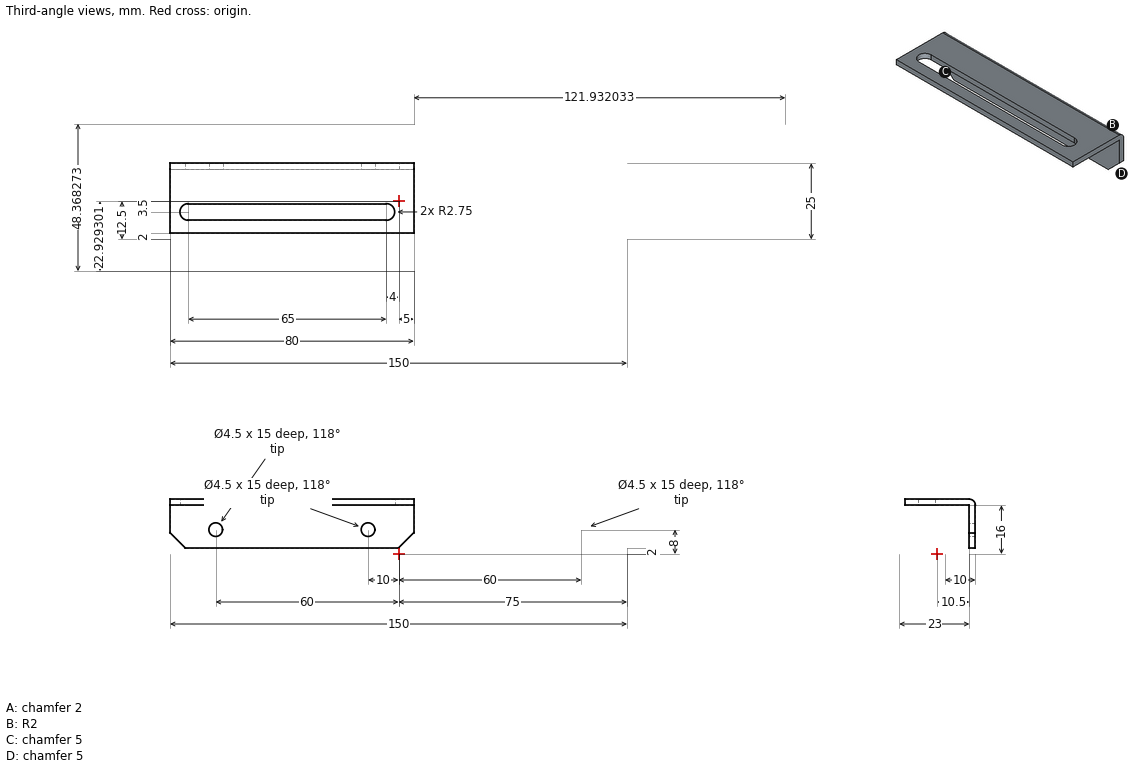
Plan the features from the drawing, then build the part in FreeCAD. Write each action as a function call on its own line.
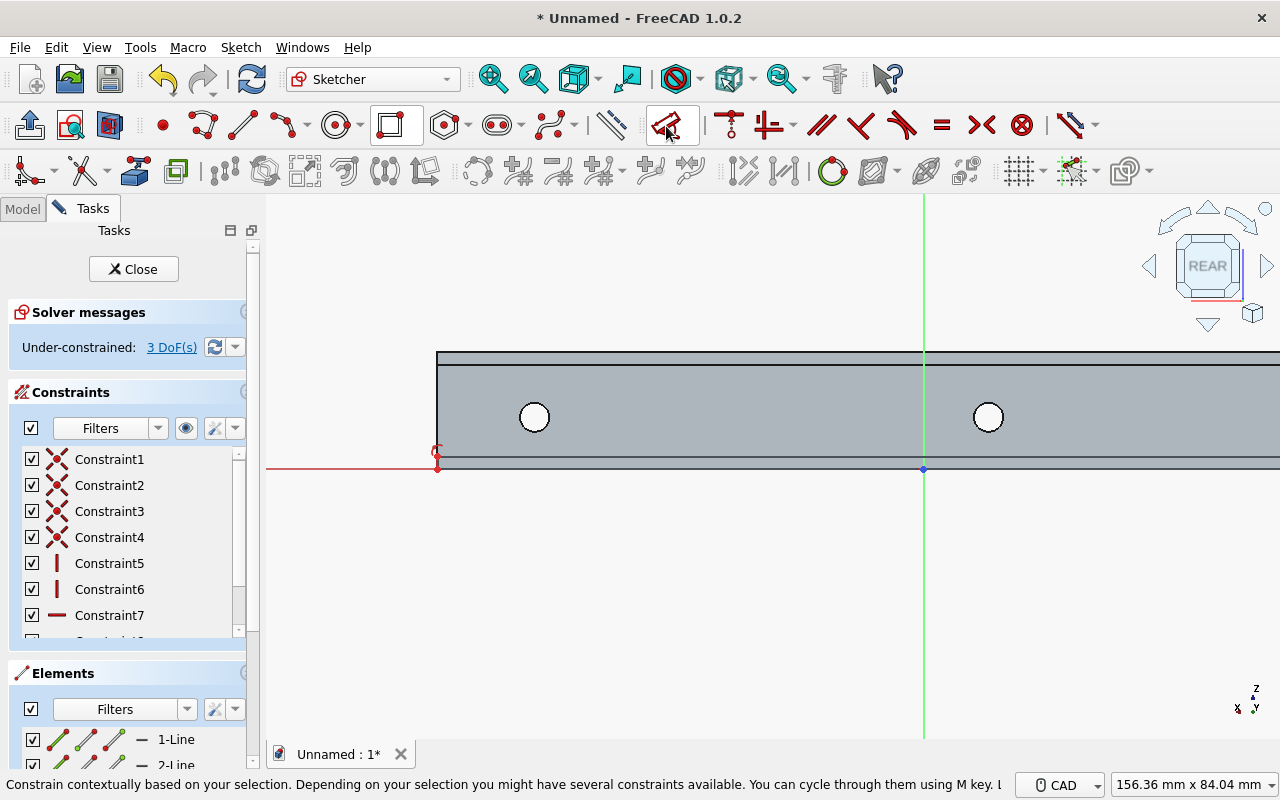
scroll(438, 463, up, 6)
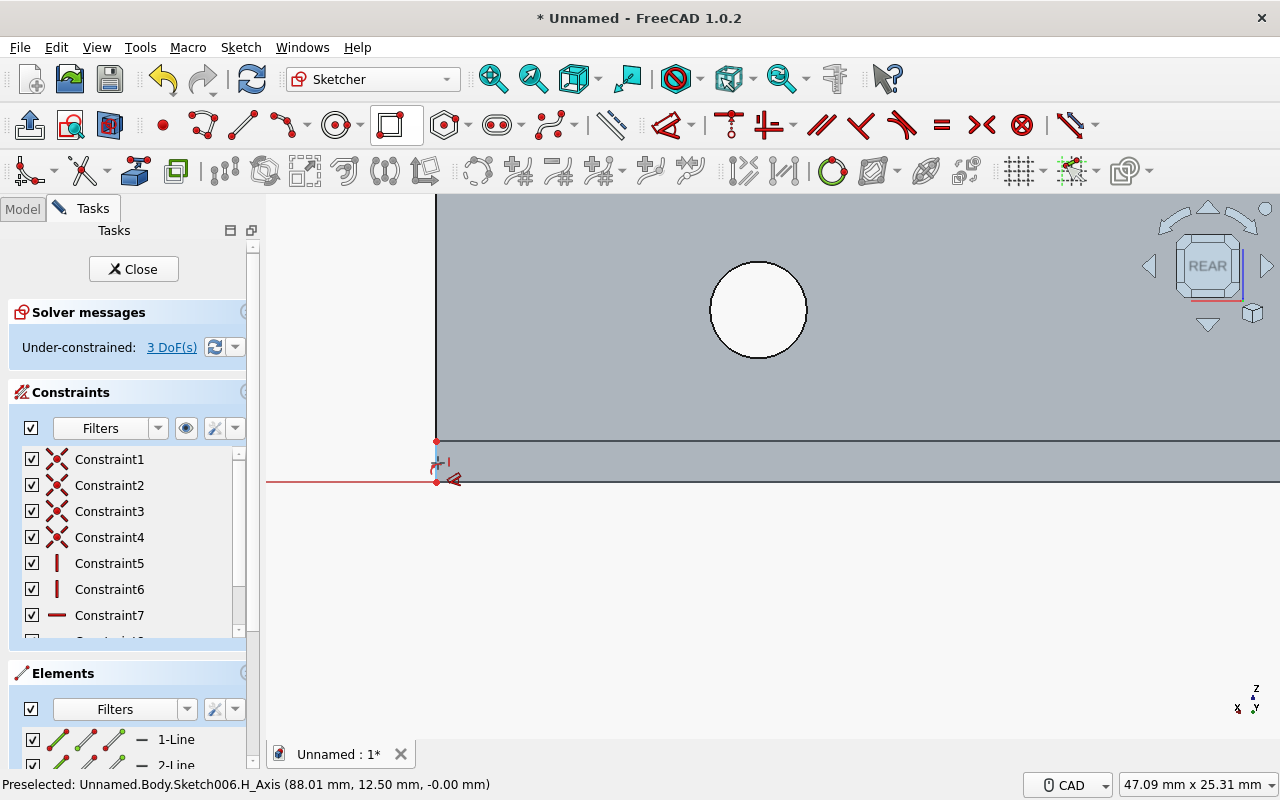
click(436, 462)
click(402, 462)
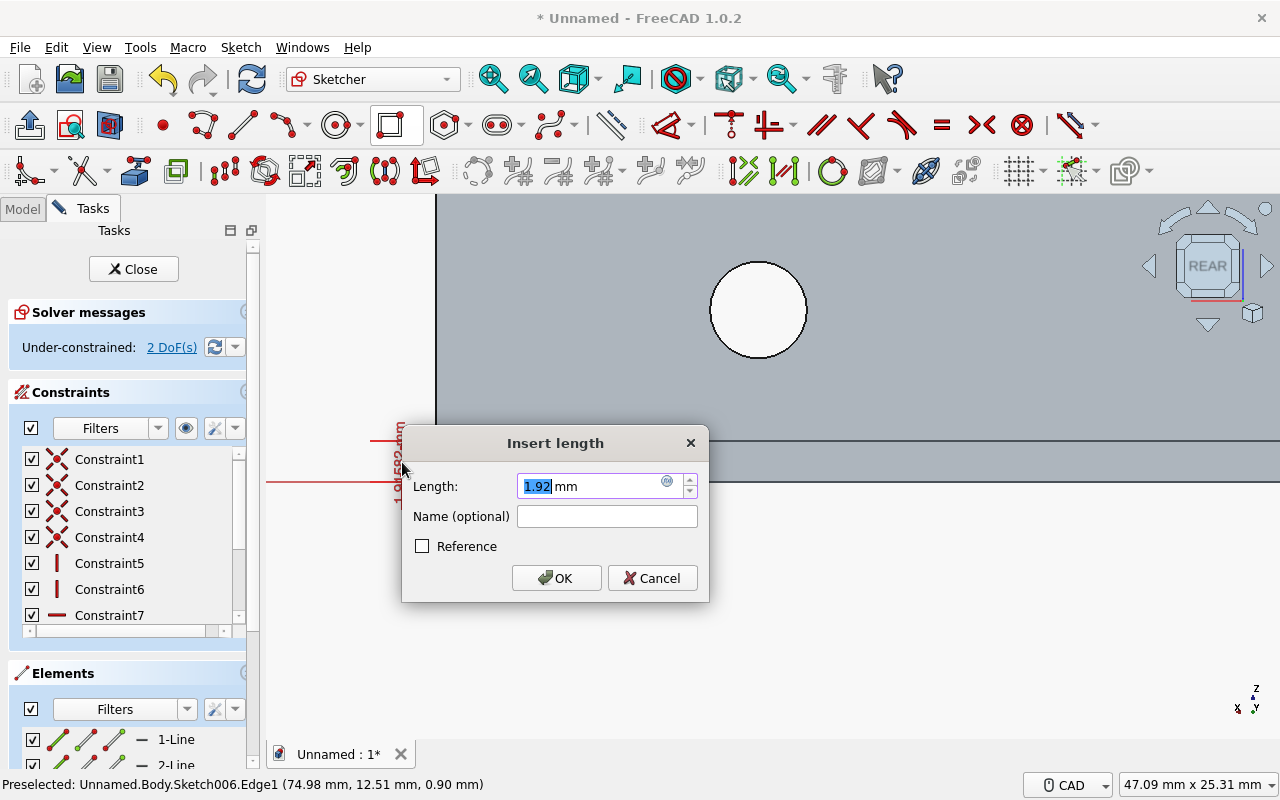
text(2)
key(Return)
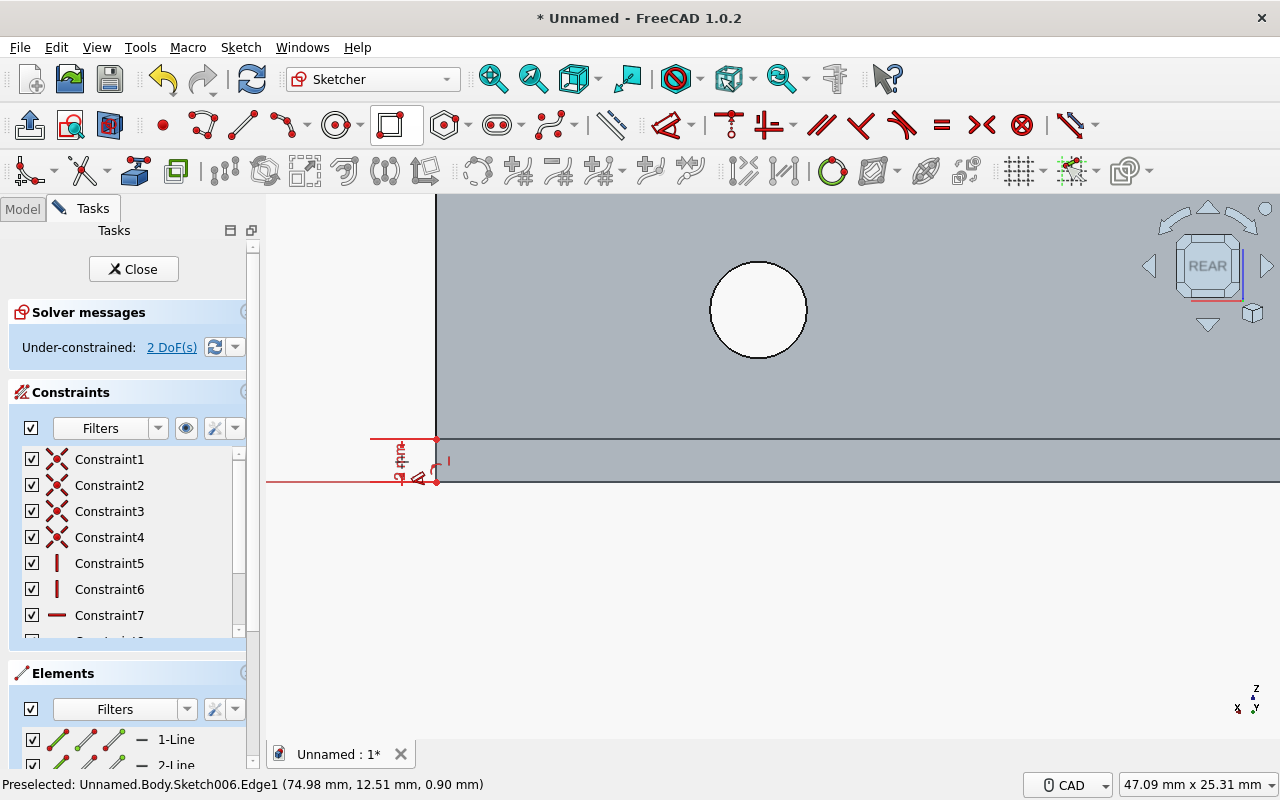
scroll(438, 468, down, 9)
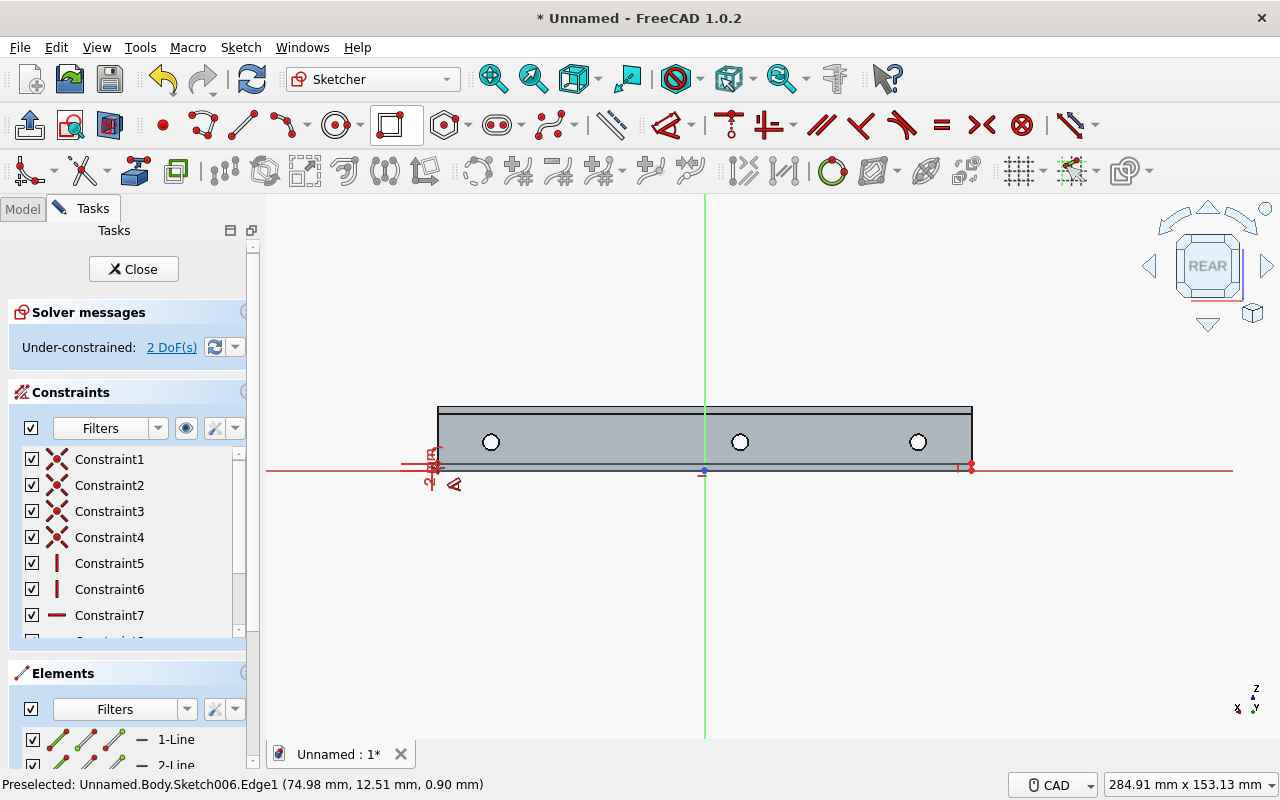
scroll(545, 471, up, 4)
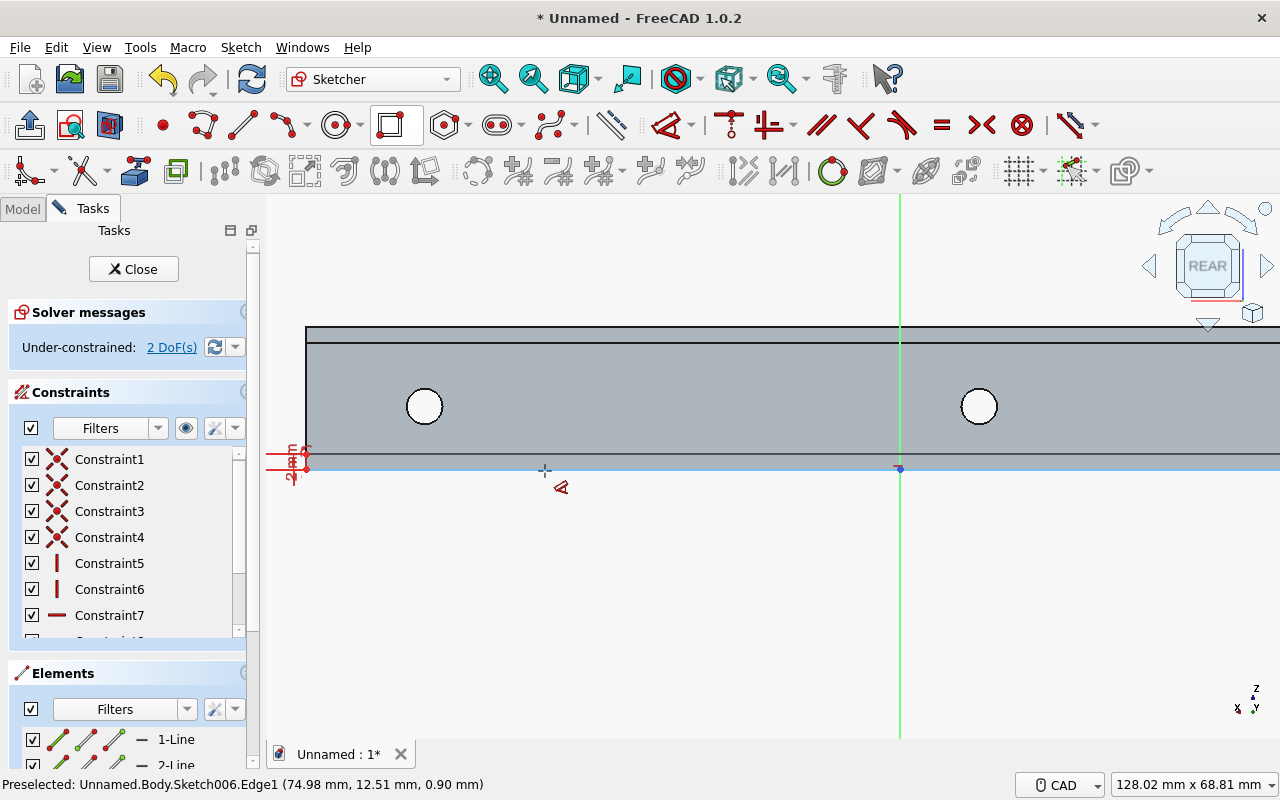
click(544, 470)
click(711, 504)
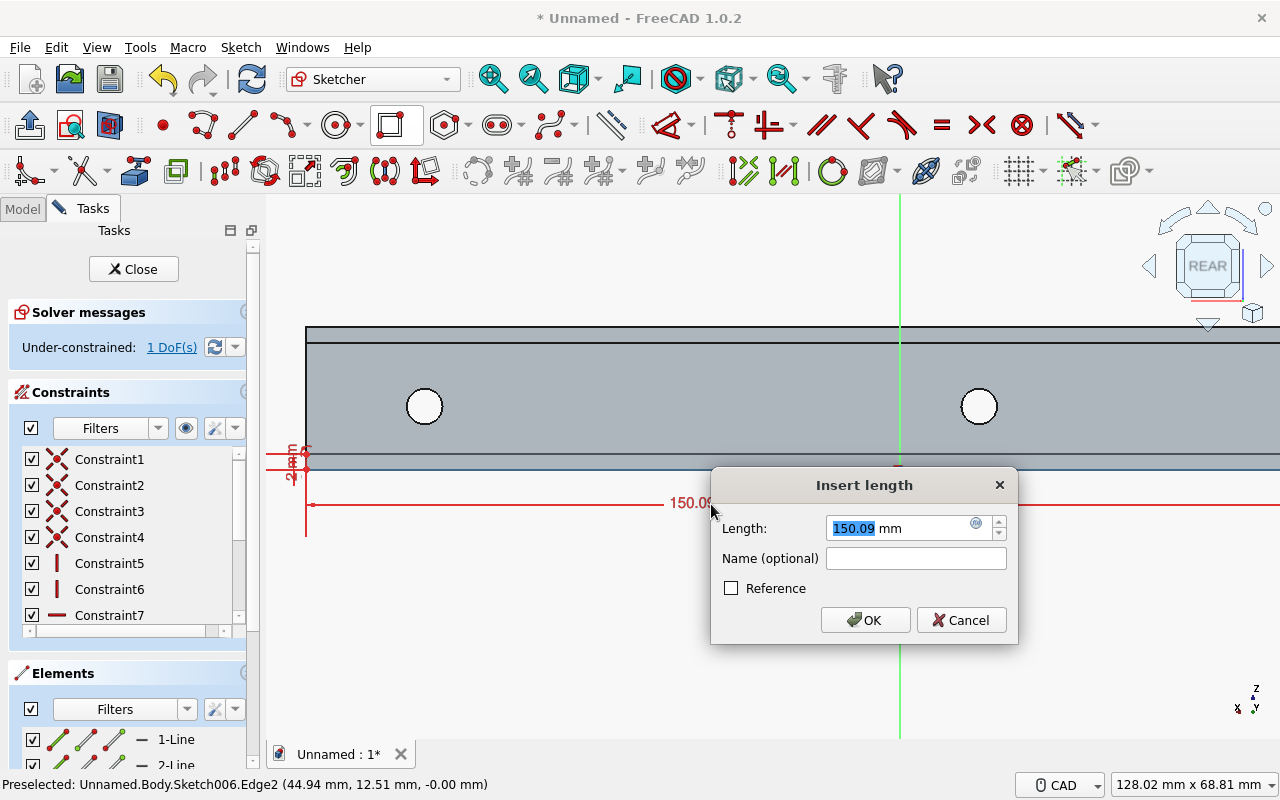
text(150)
key(Return)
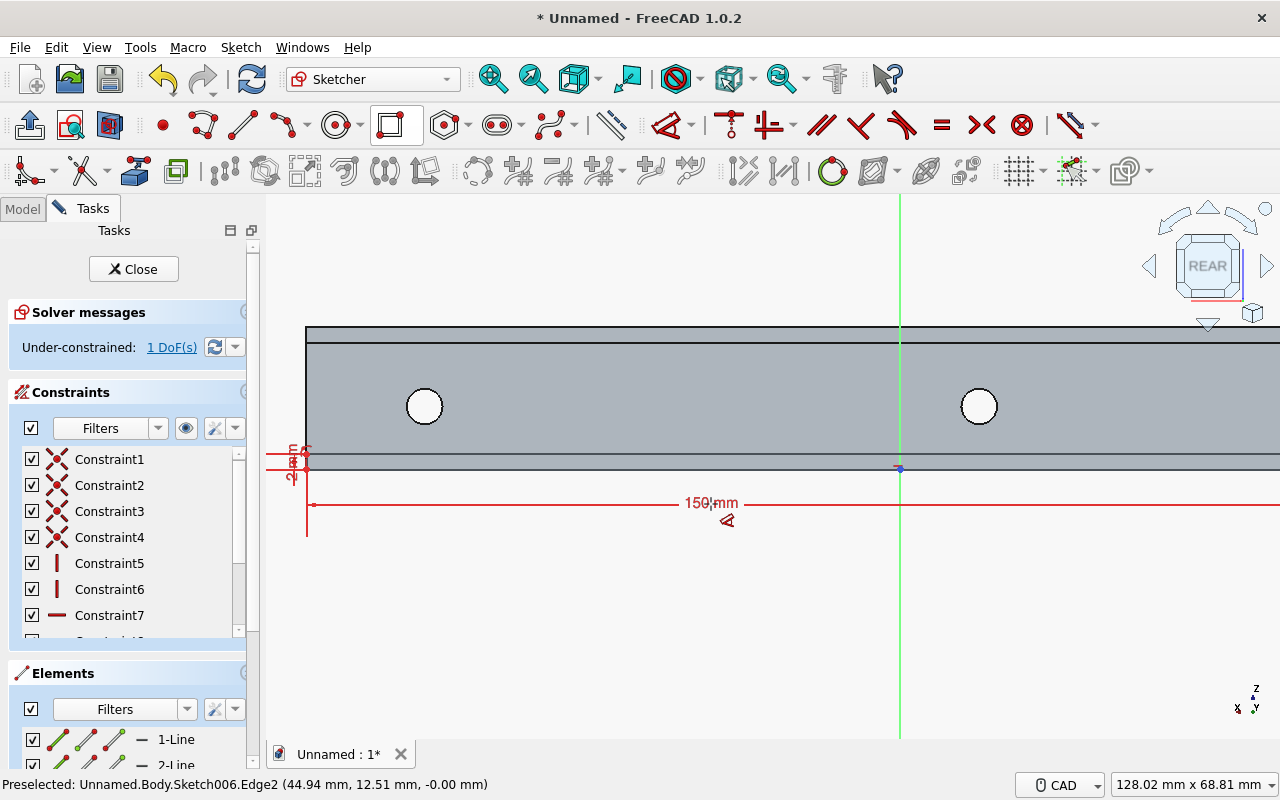
click(307, 454)
click(603, 504)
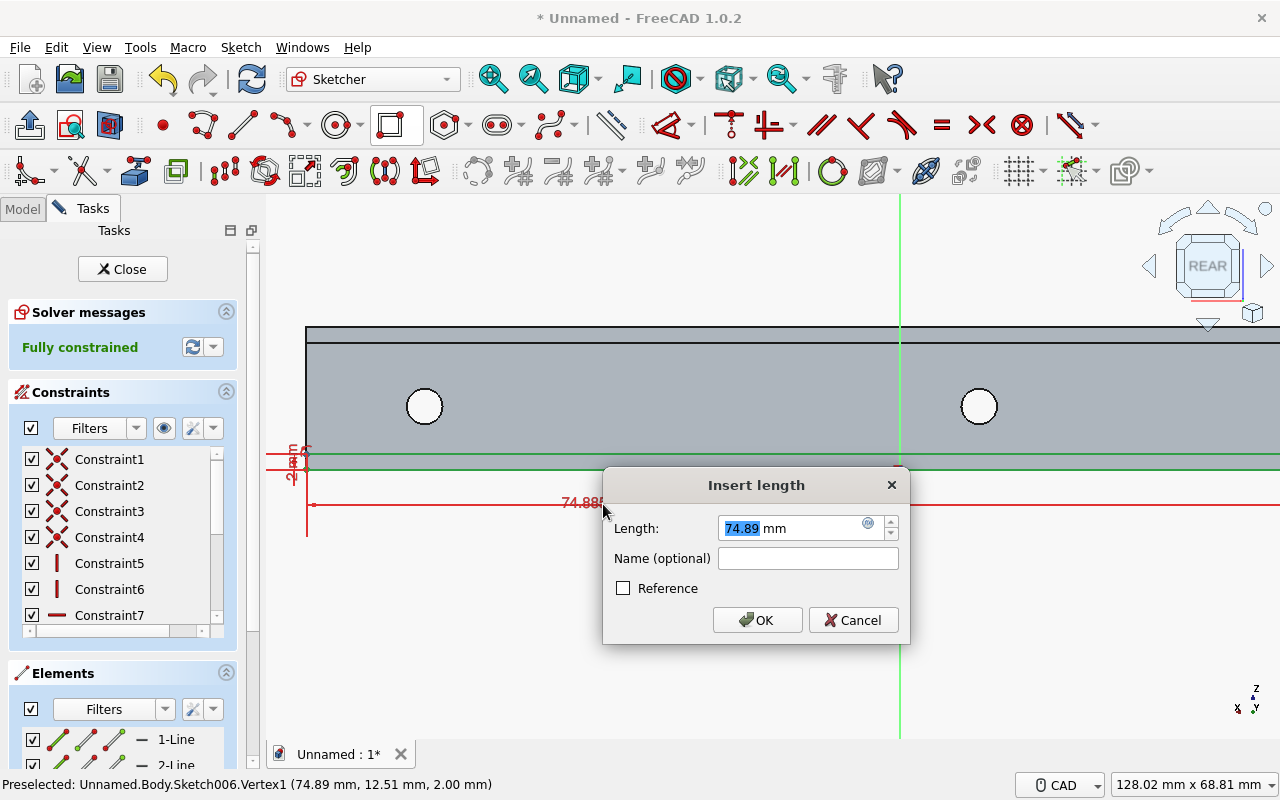
text(75)
key(Return)
key(Escape)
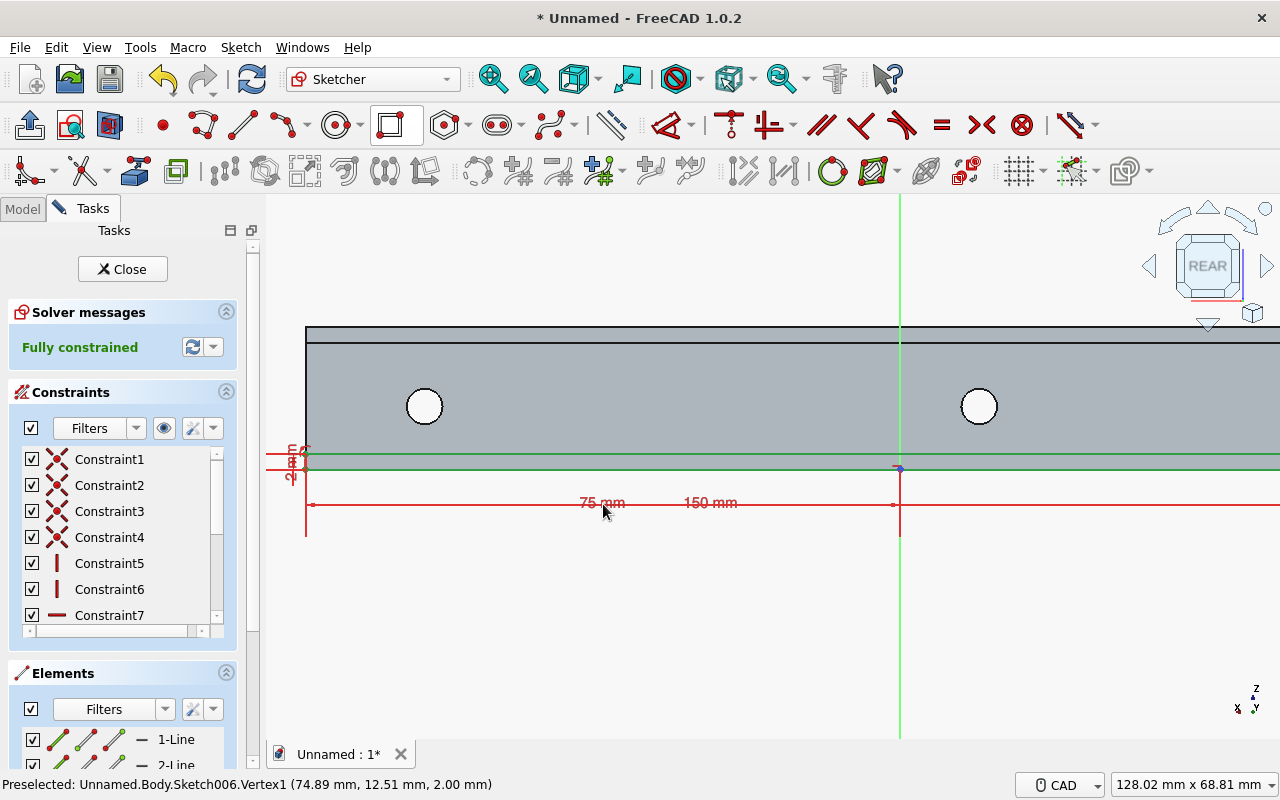
click(123, 269)